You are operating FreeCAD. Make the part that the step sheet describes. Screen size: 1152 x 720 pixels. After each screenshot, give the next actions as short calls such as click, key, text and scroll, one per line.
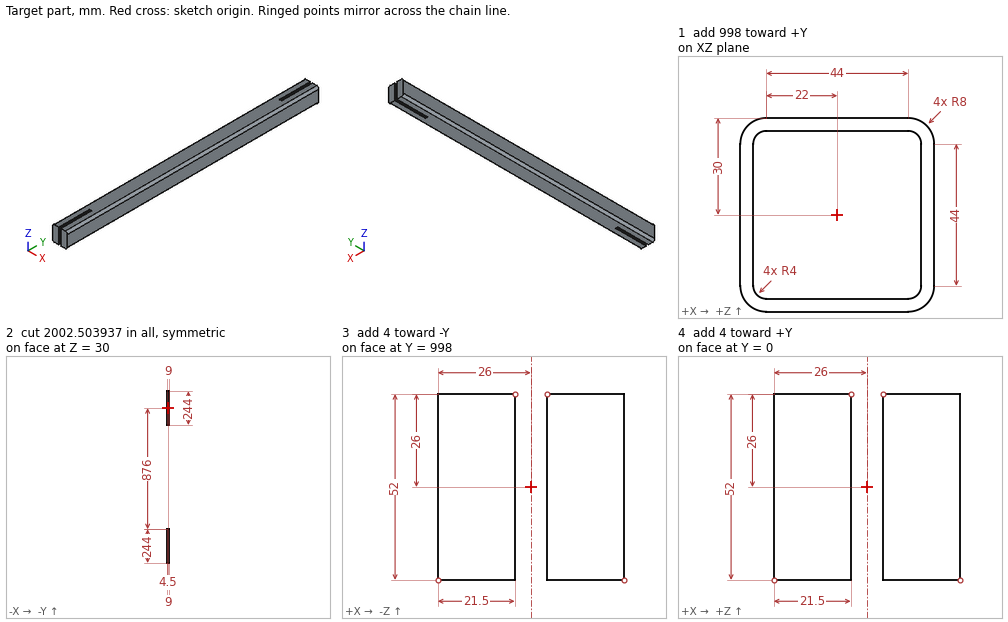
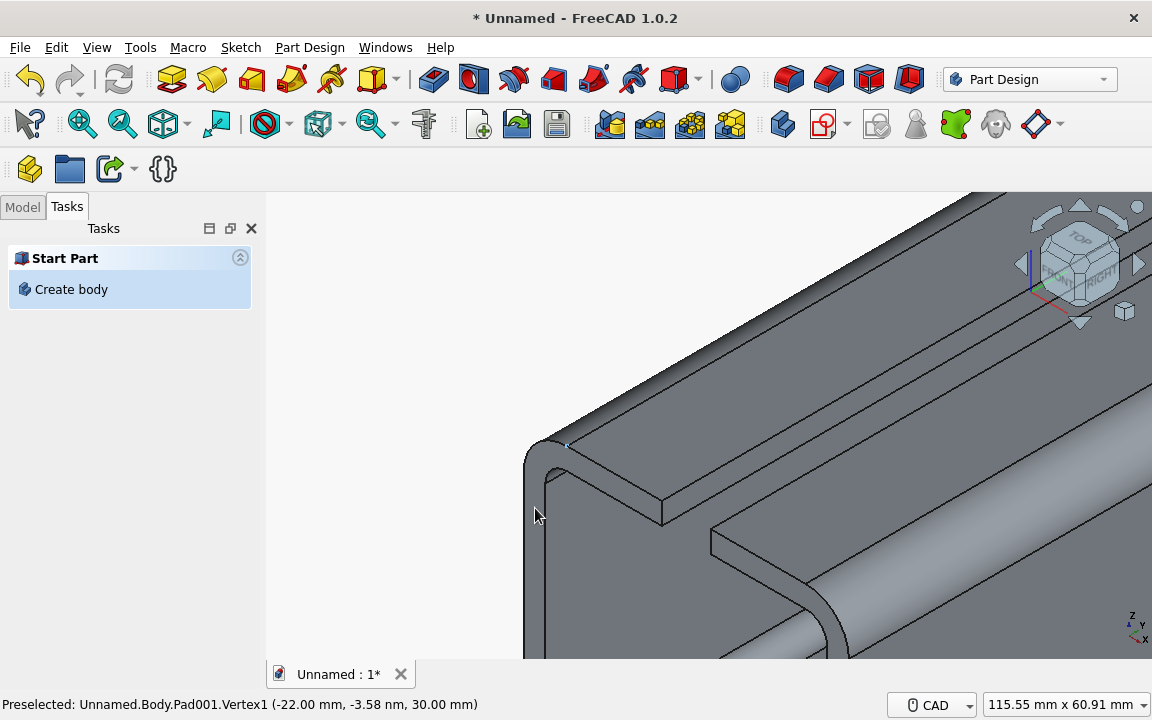
click(533, 506)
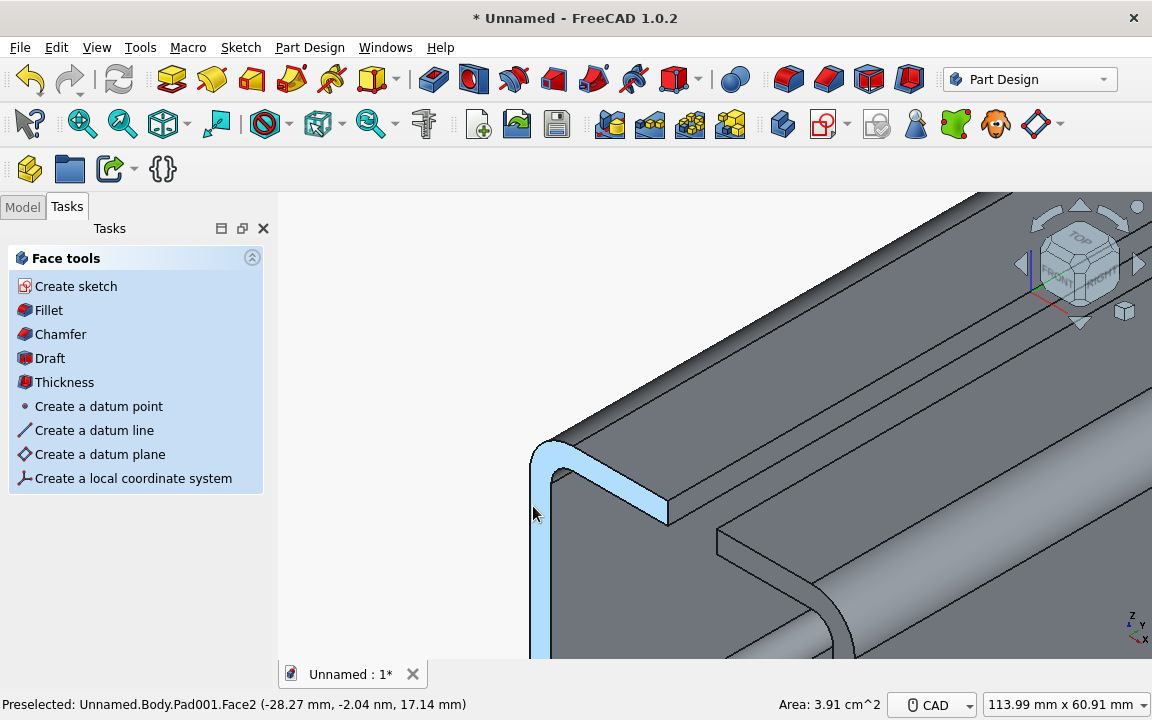
click(824, 124)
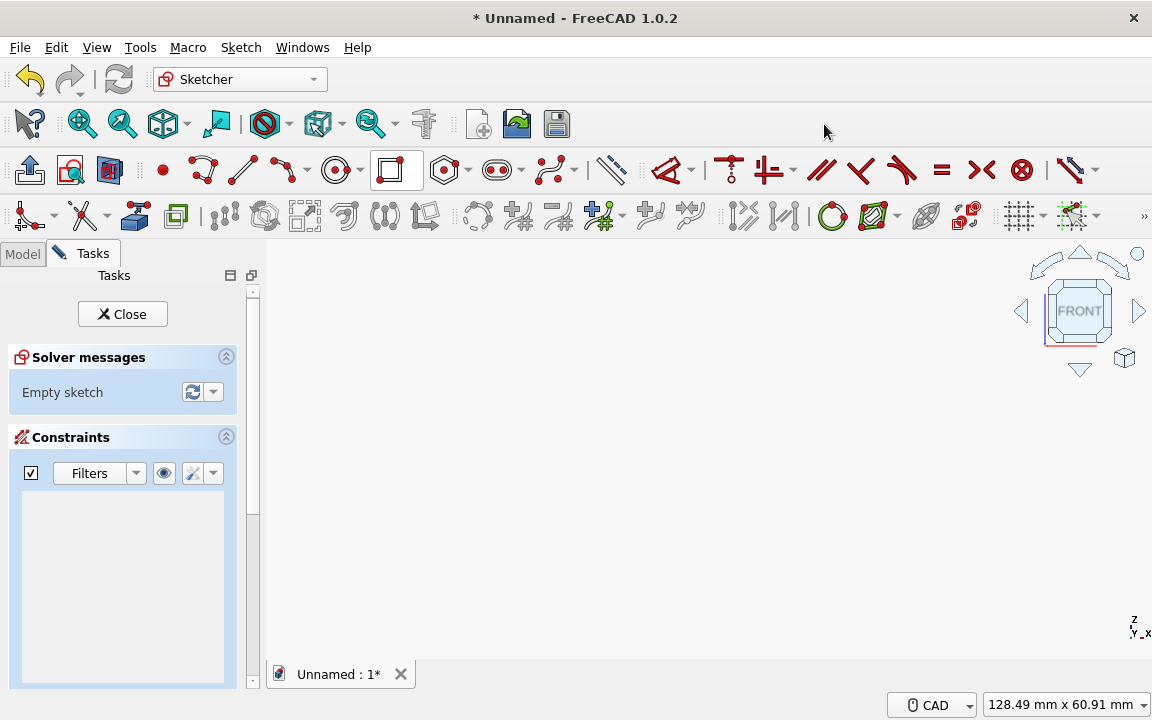
scroll(640, 449, down, 5)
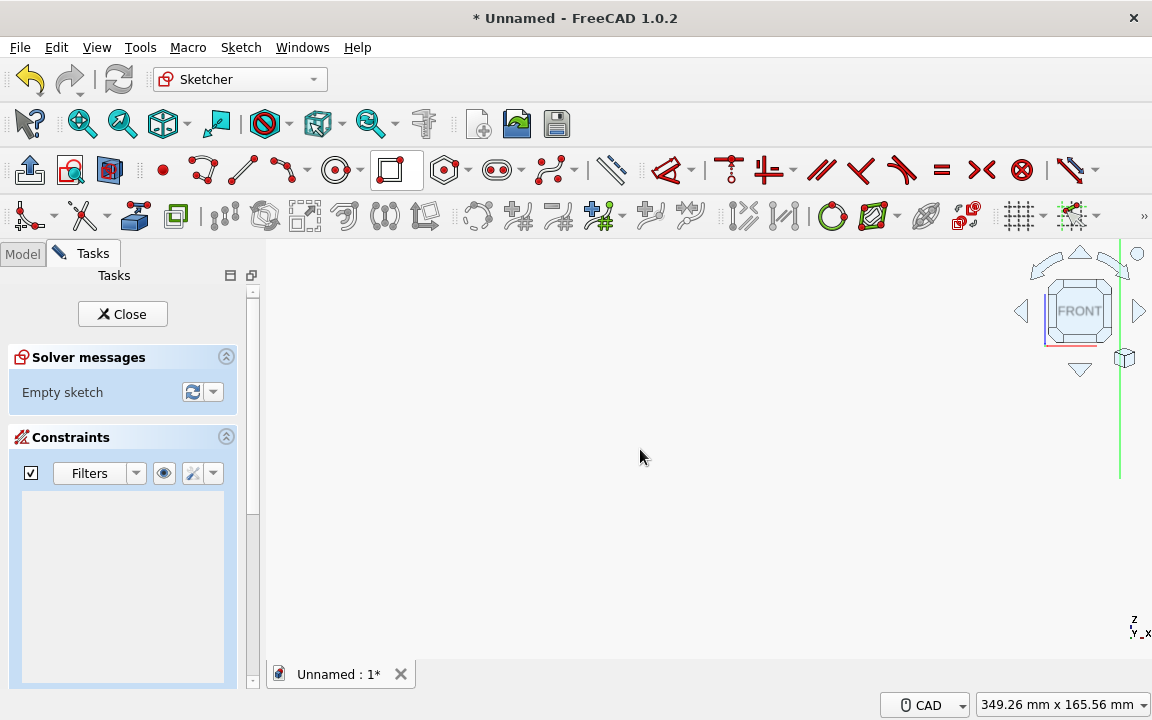
scroll(640, 449, down, 5)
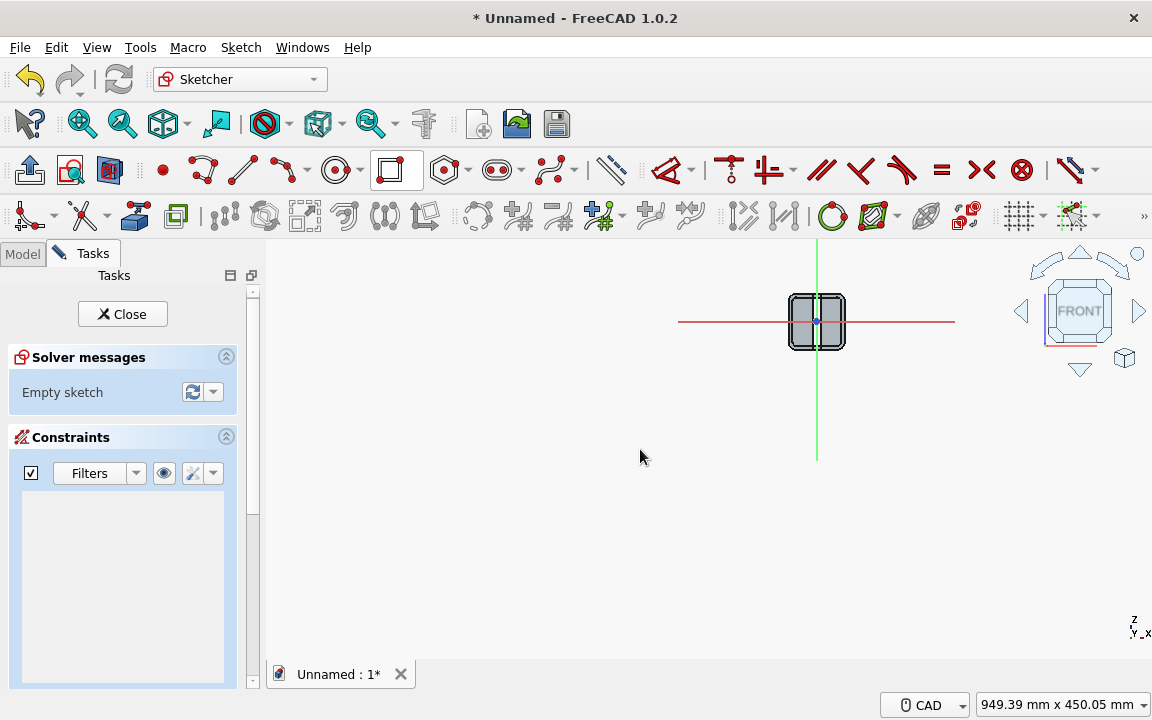
scroll(861, 290, up, 8)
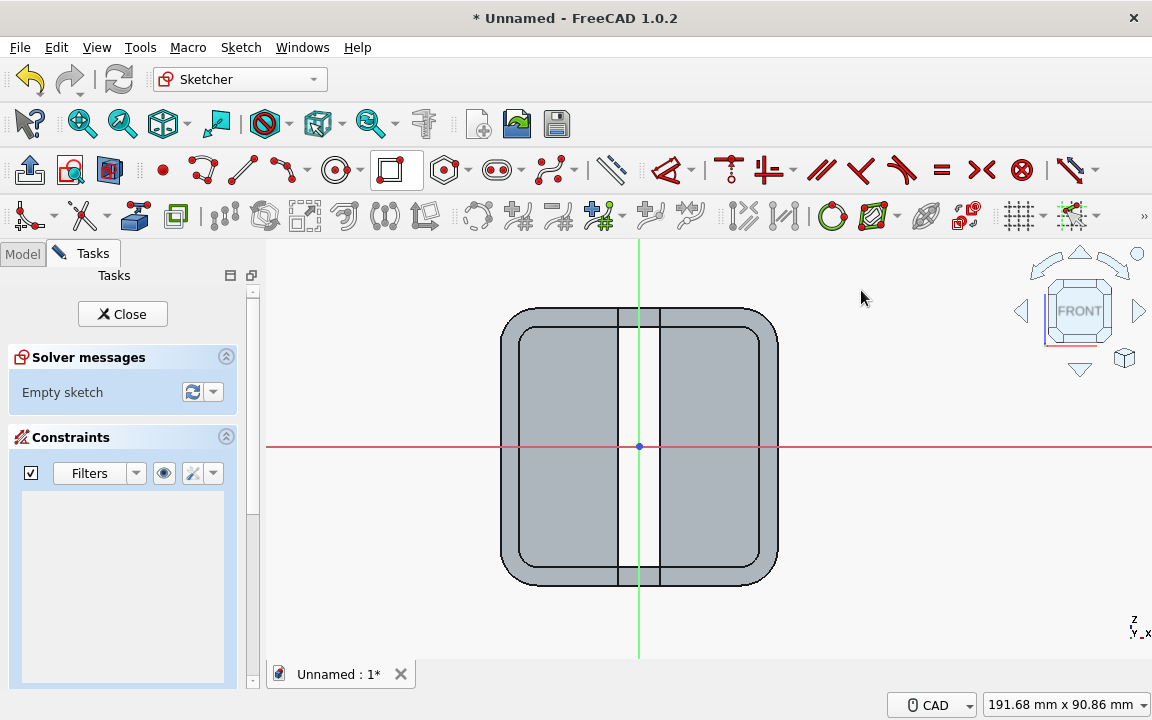
click(390, 170)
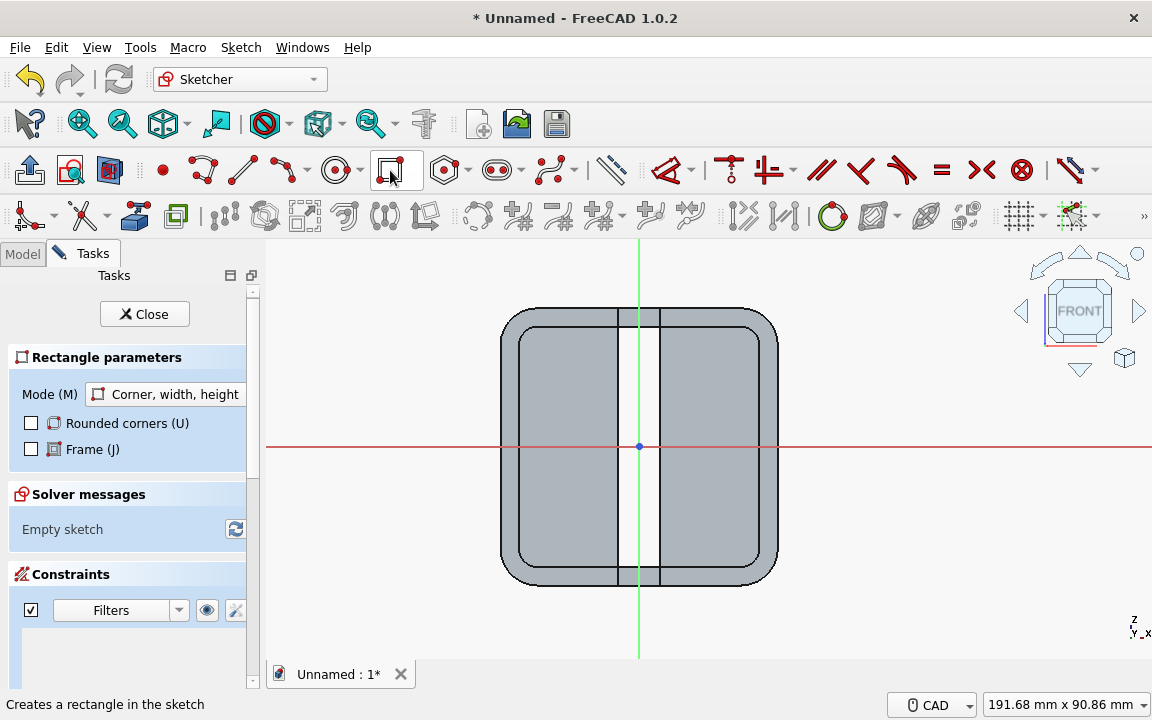
click(519, 327)
click(618, 567)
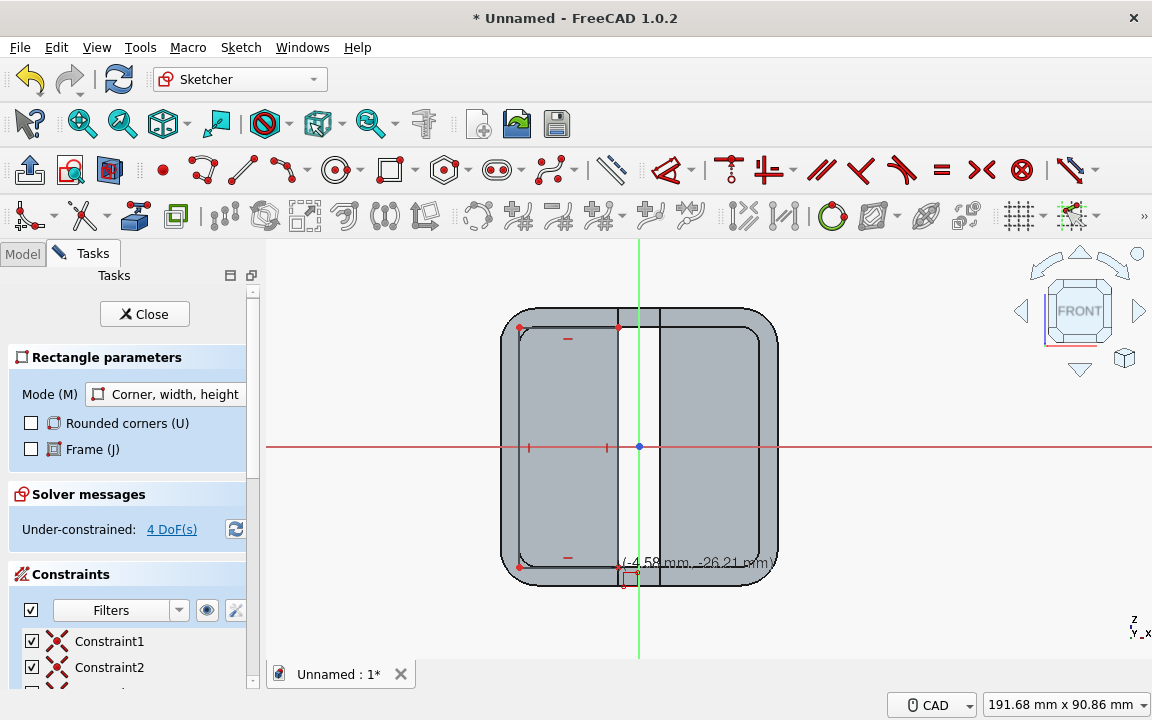
click(660, 327)
click(759, 567)
key(Escape)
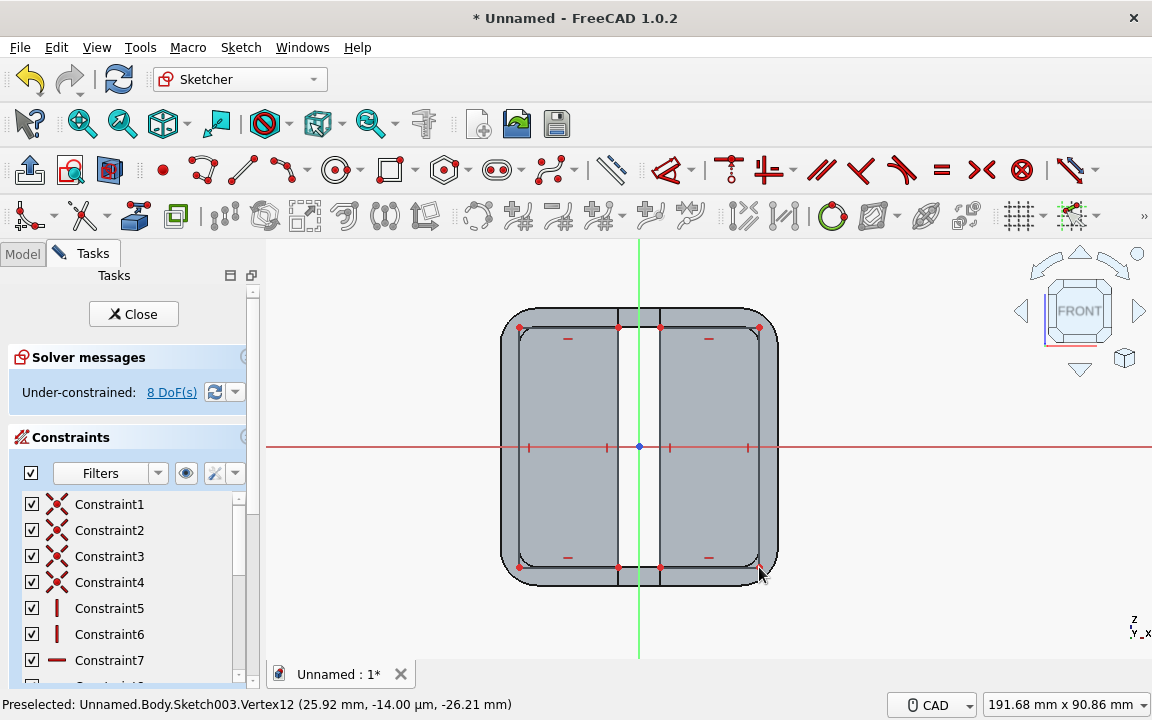
click(618, 328)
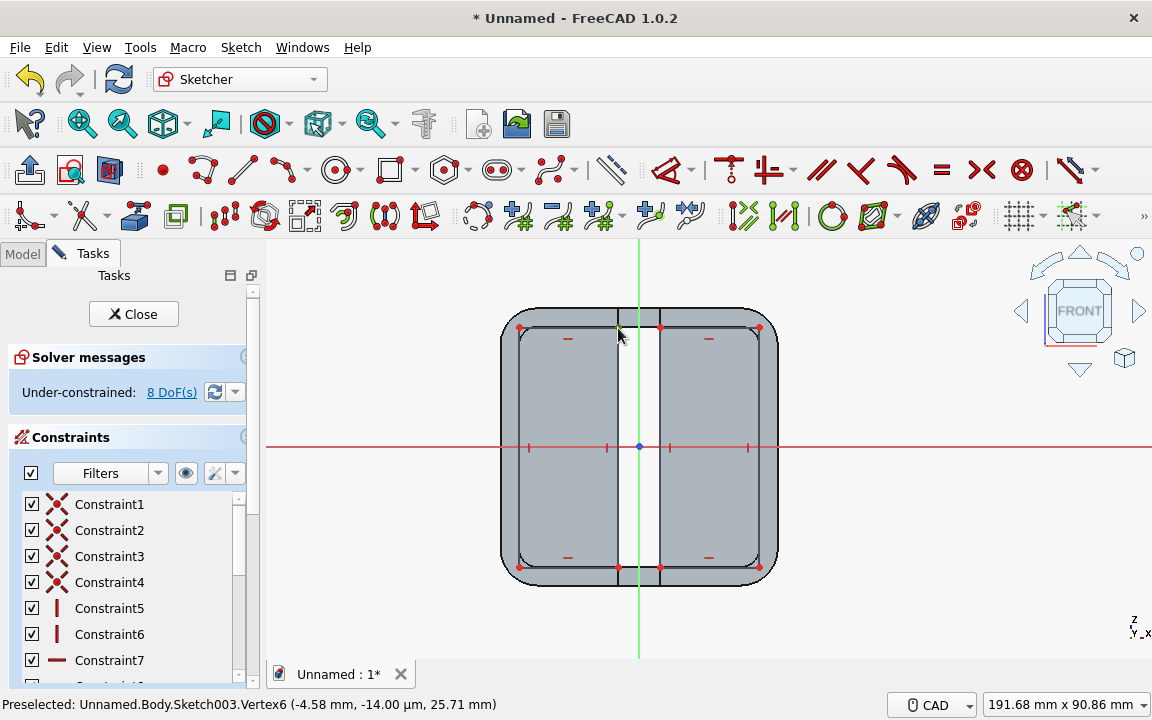
click(660, 328)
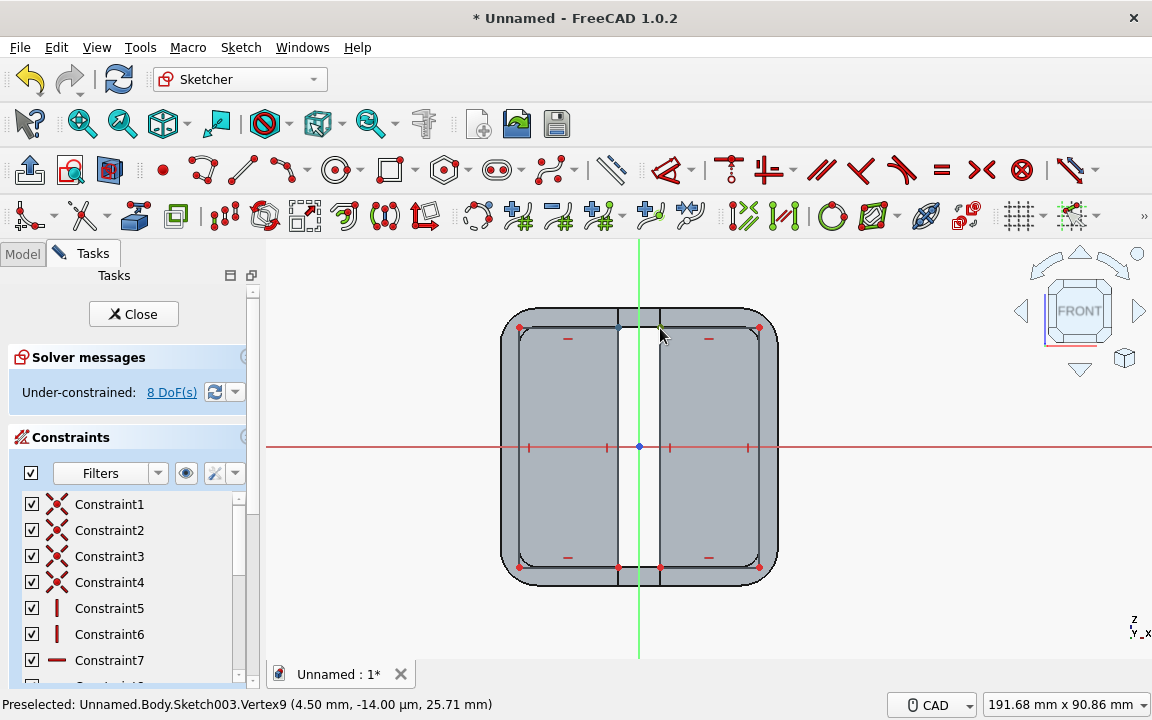
click(639, 605)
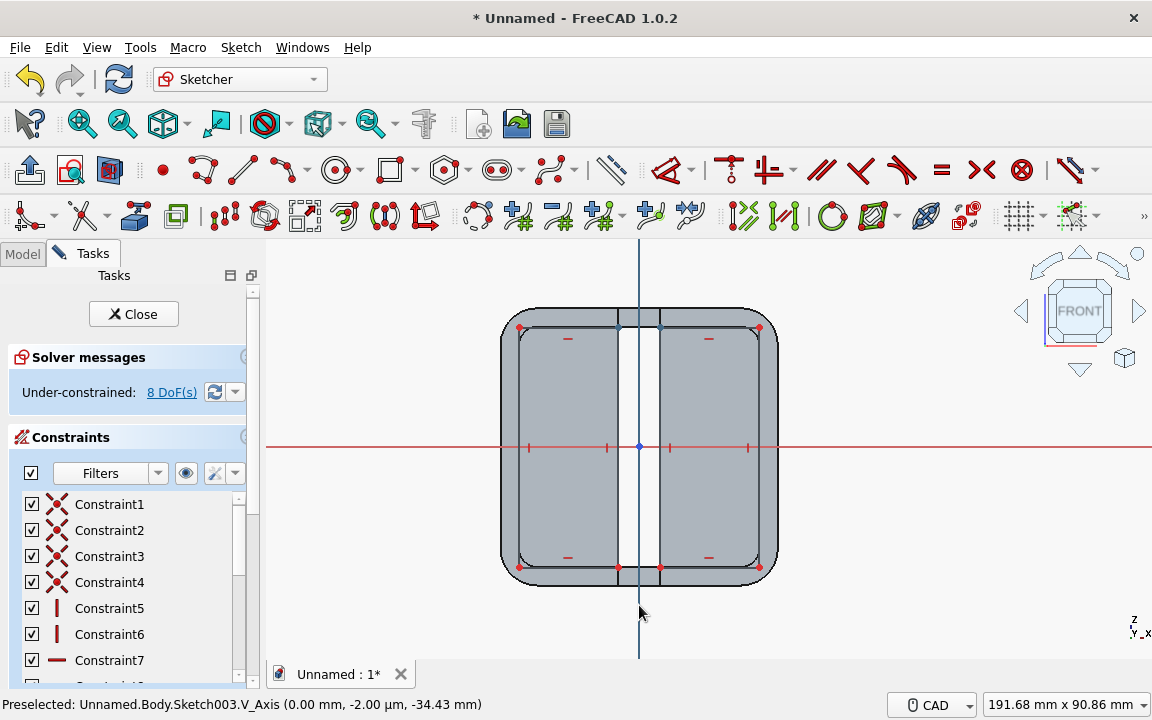
click(982, 170)